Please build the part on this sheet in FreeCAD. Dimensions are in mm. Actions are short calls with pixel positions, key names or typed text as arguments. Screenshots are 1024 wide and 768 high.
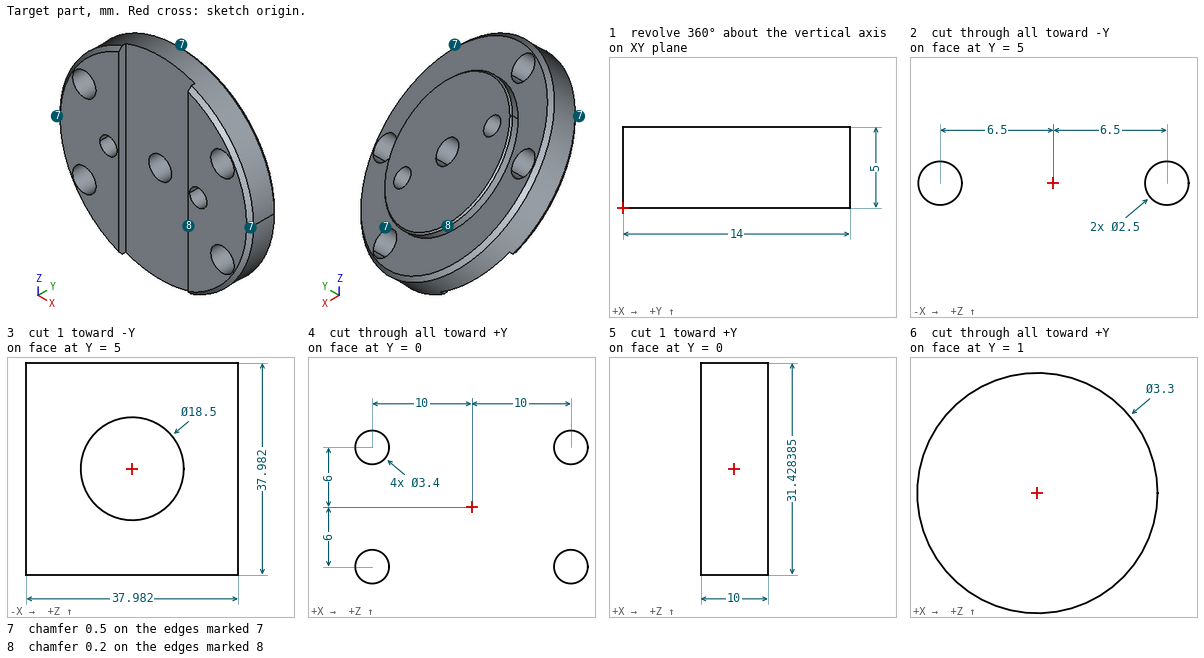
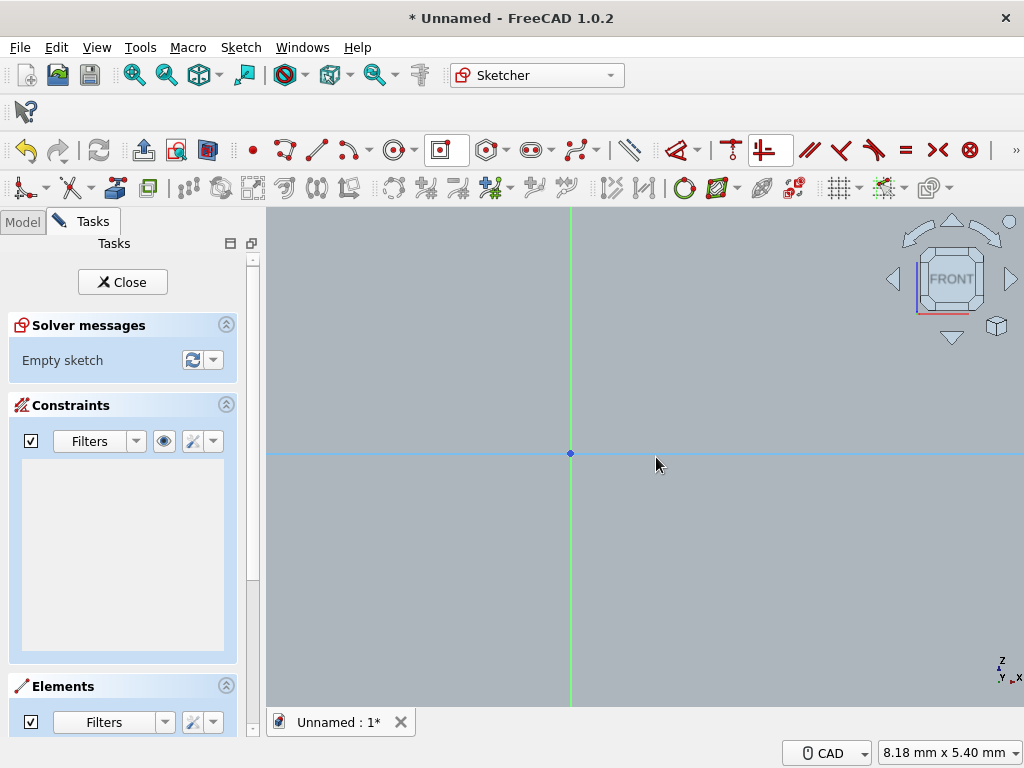
key(g)
key(c)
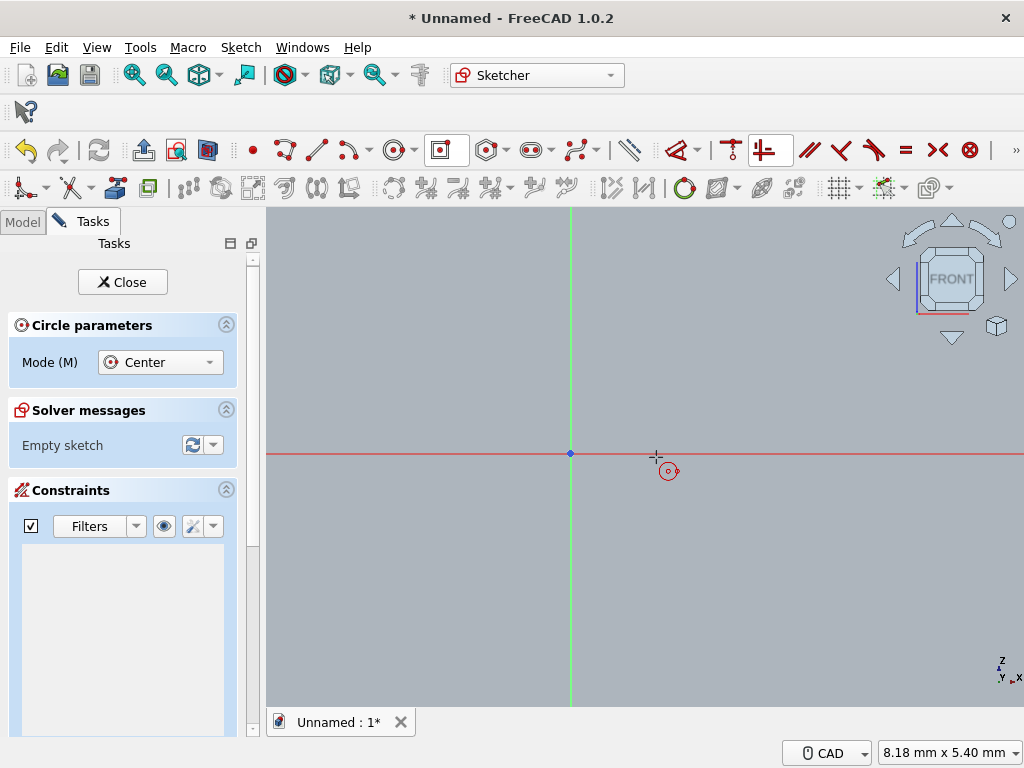
click(571, 454)
click(679, 346)
key(Escape)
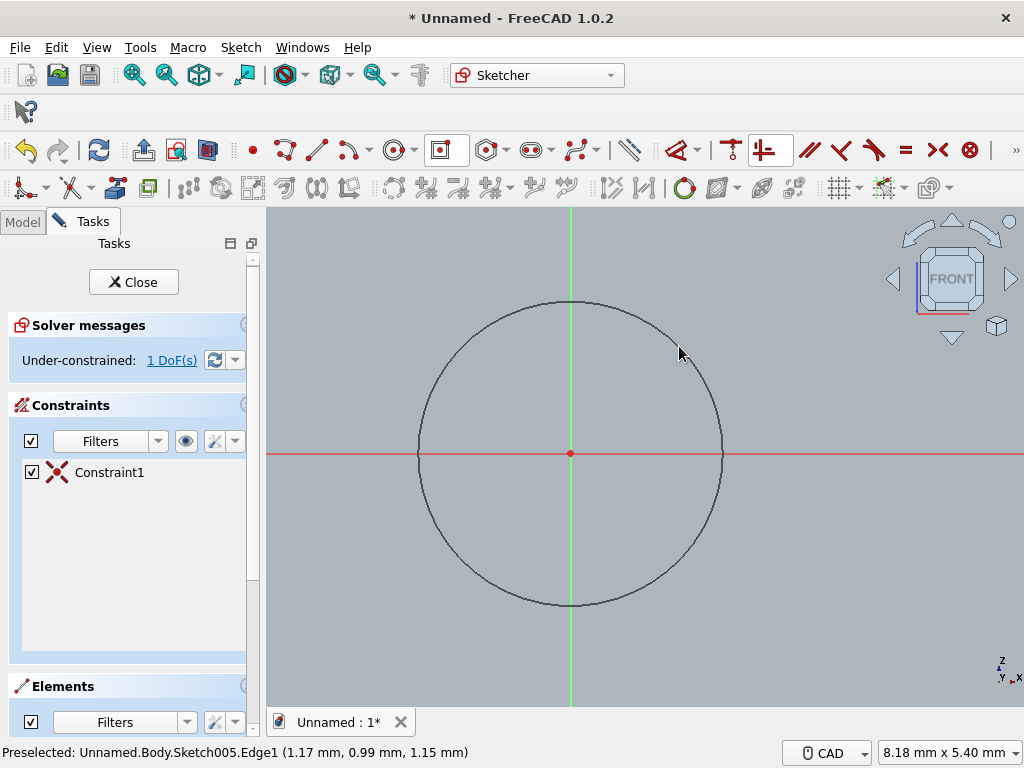
key(d)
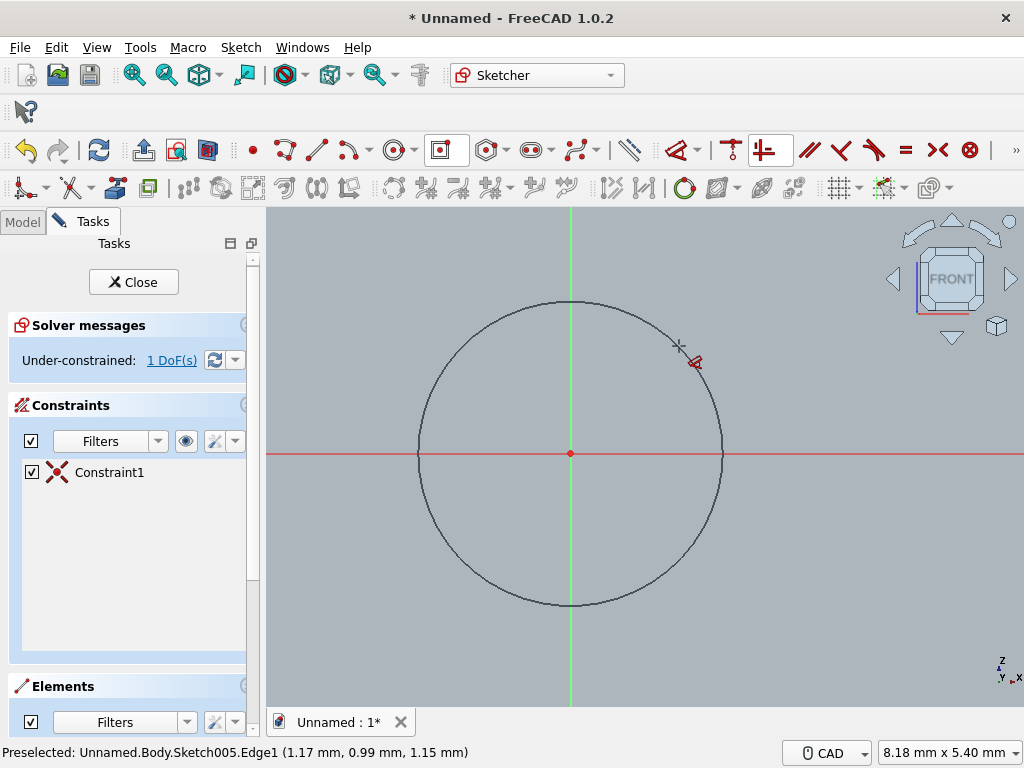
click(678, 346)
click(701, 323)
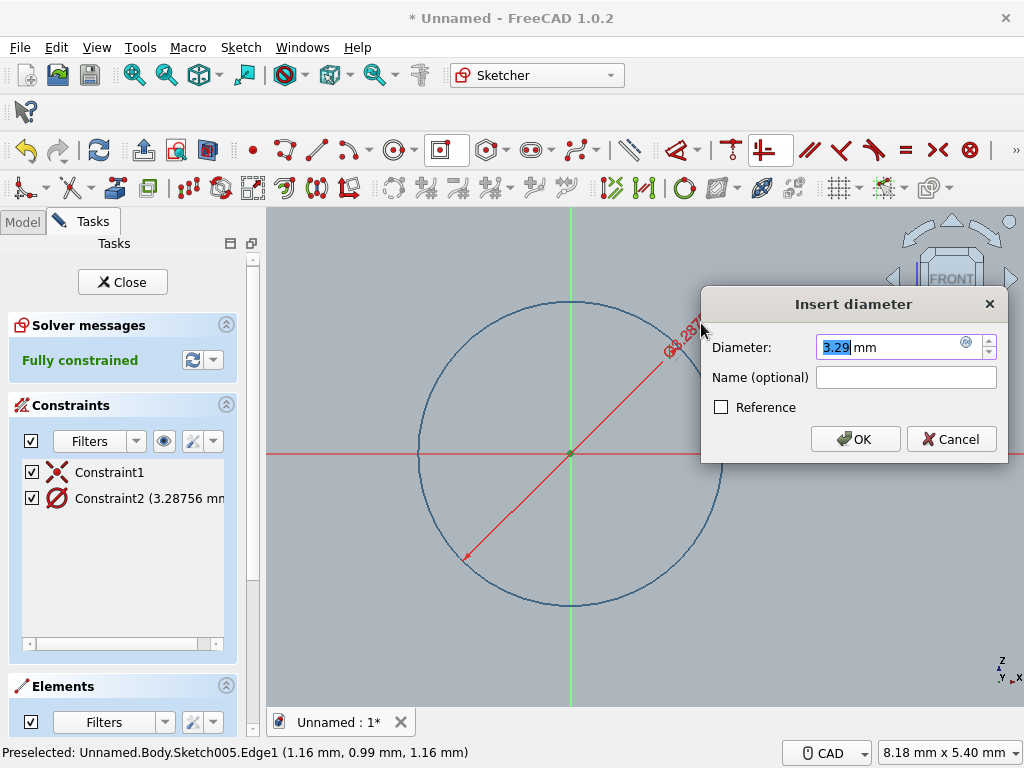
text(3.3)
key(Return)
key(Escape)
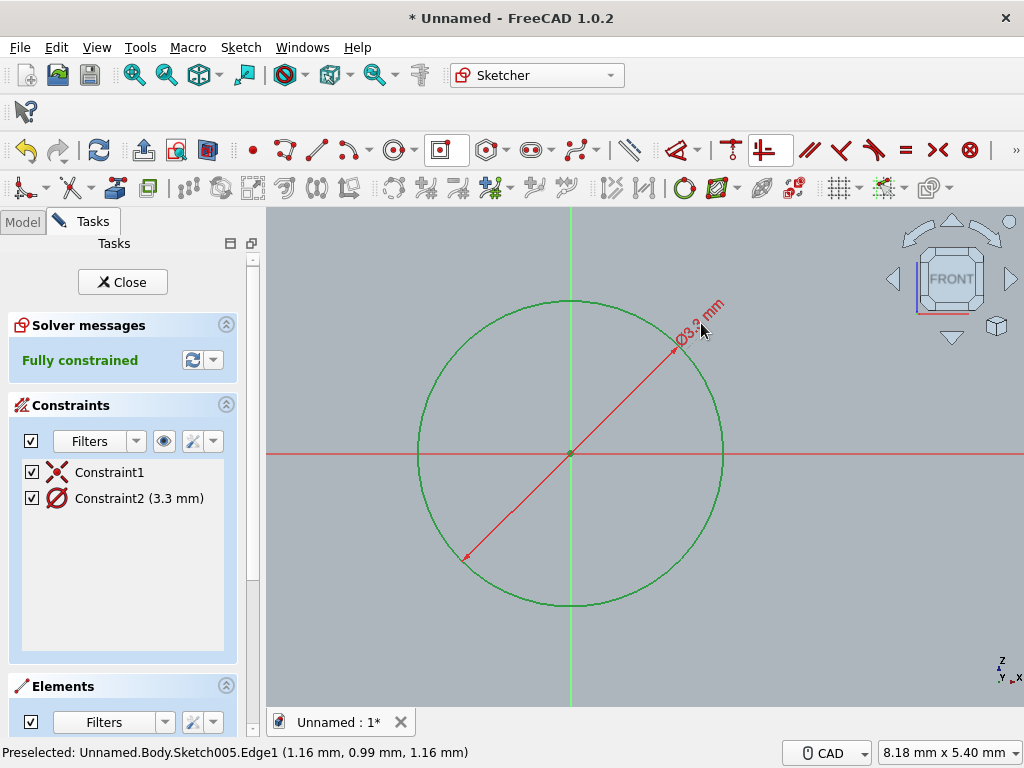
click(123, 282)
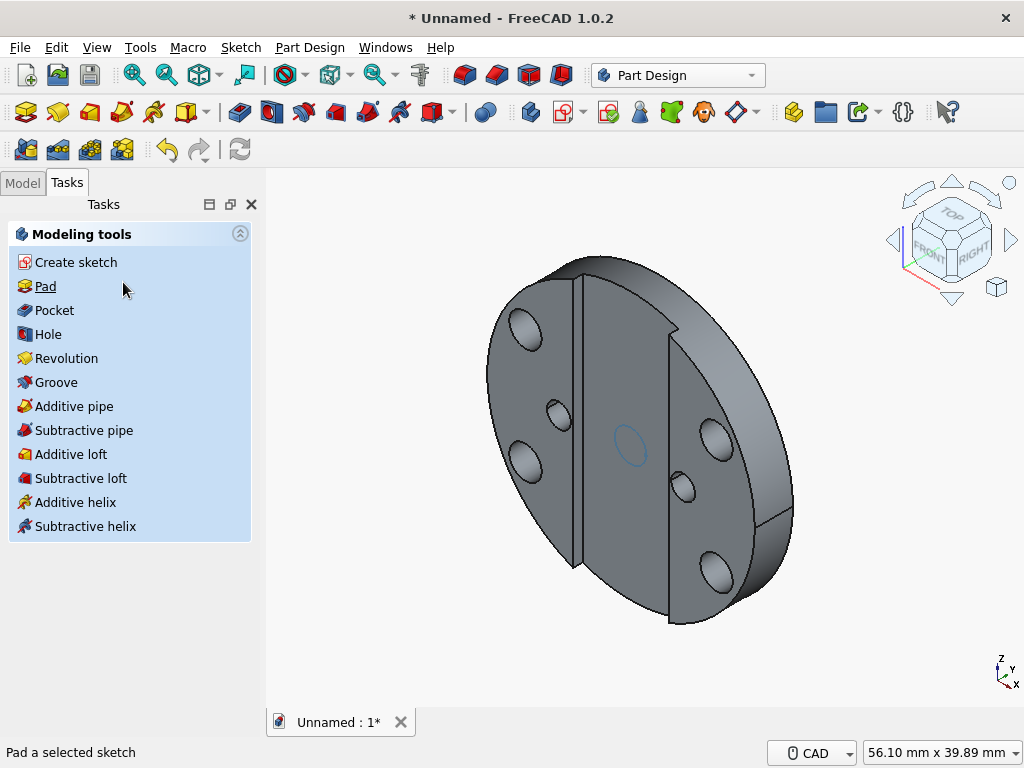
click(240, 112)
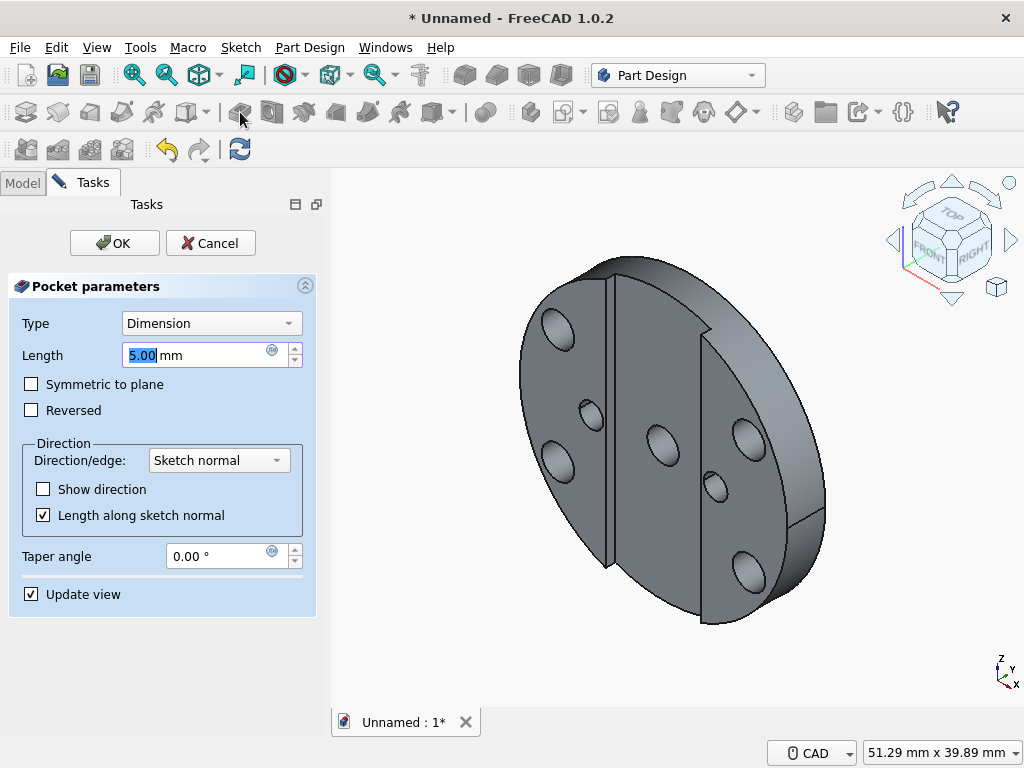
click(212, 324)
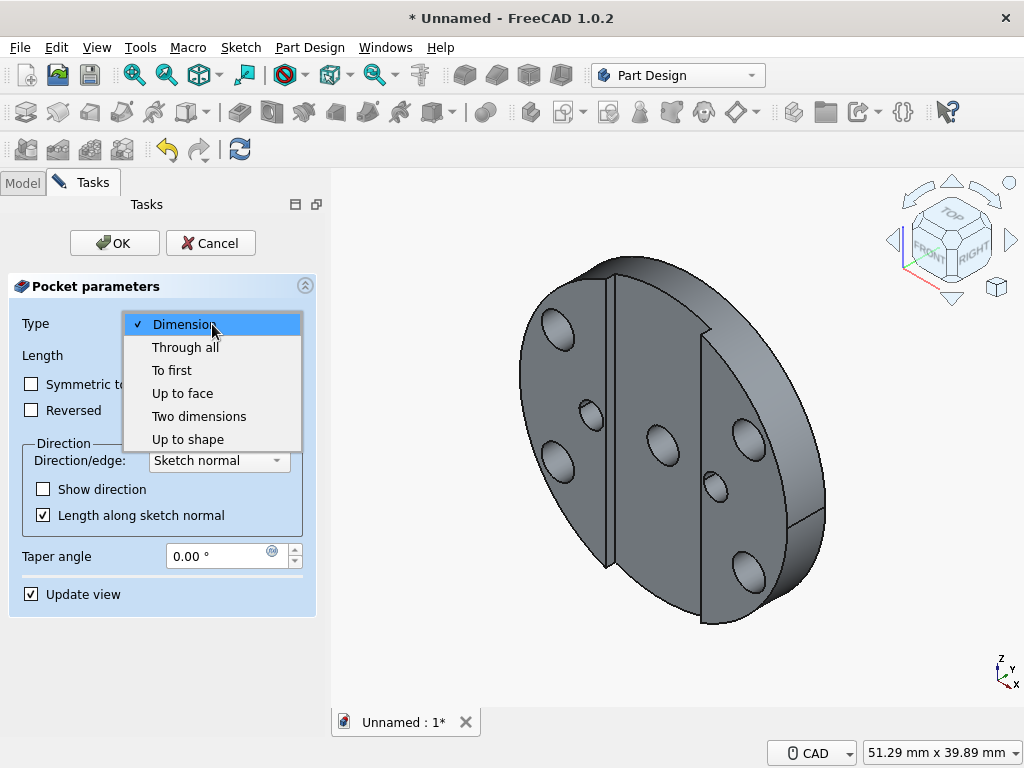
click(212, 348)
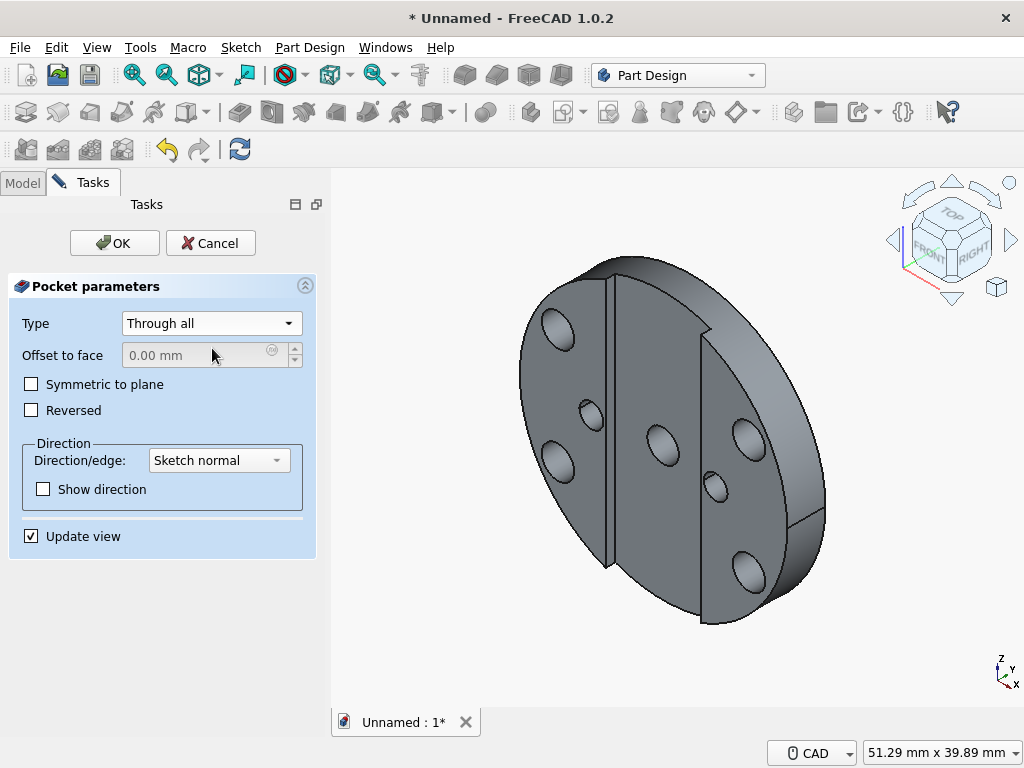
click(115, 243)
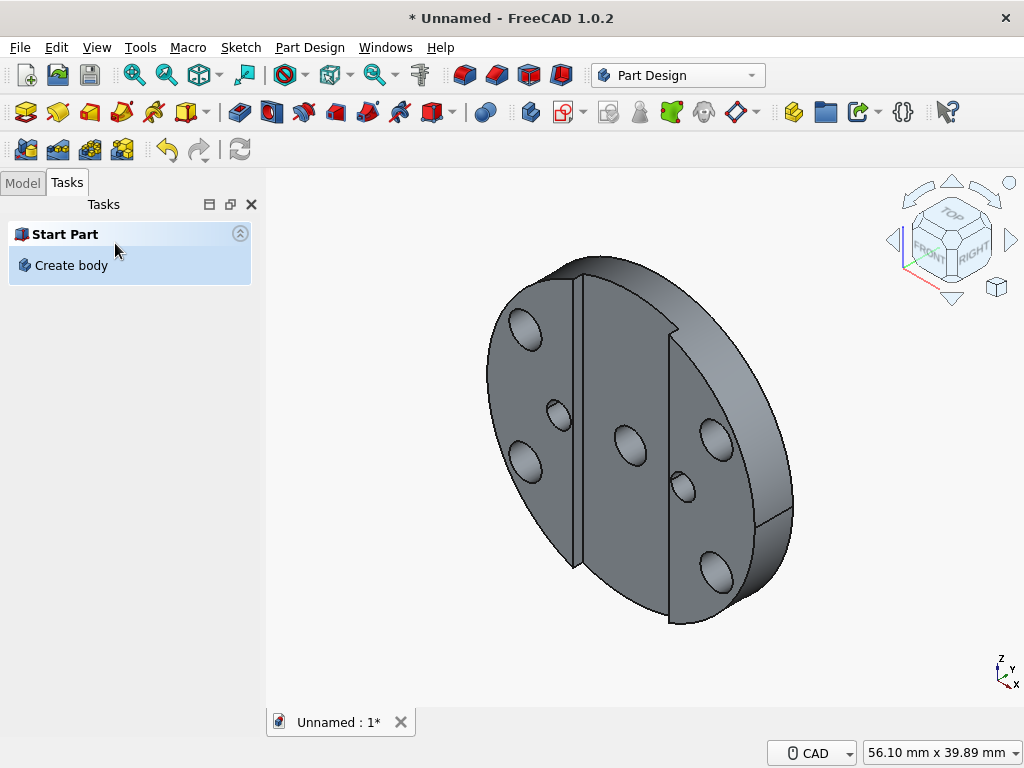
click(731, 426)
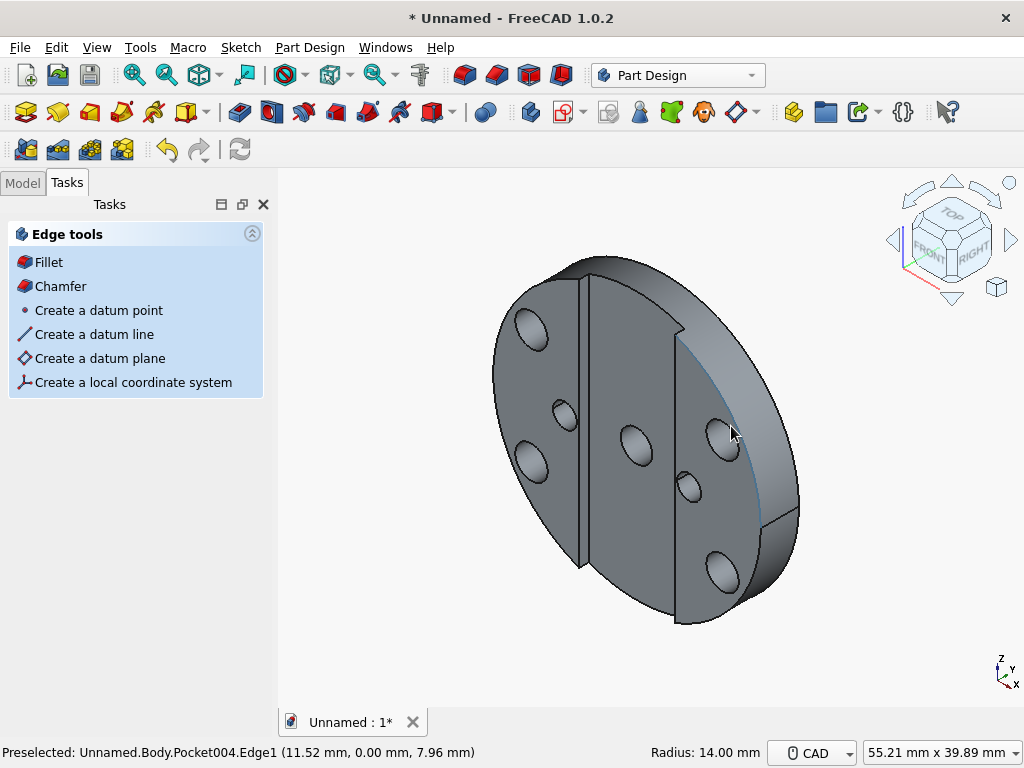
click(497, 338, ctrl)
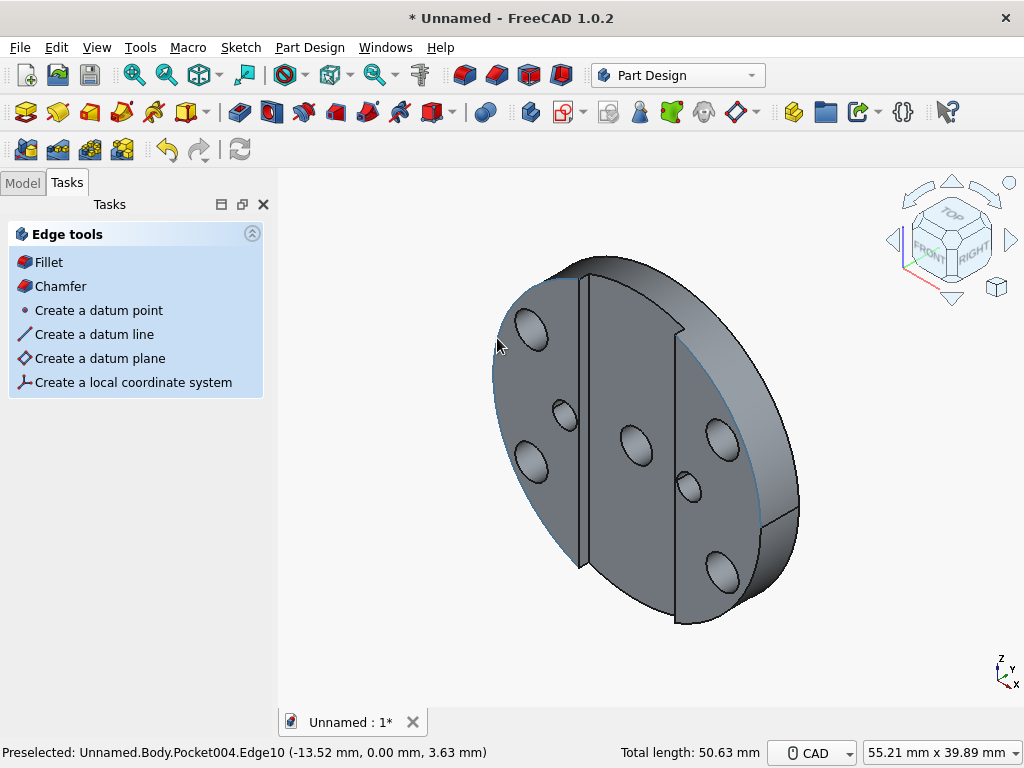
key(2)